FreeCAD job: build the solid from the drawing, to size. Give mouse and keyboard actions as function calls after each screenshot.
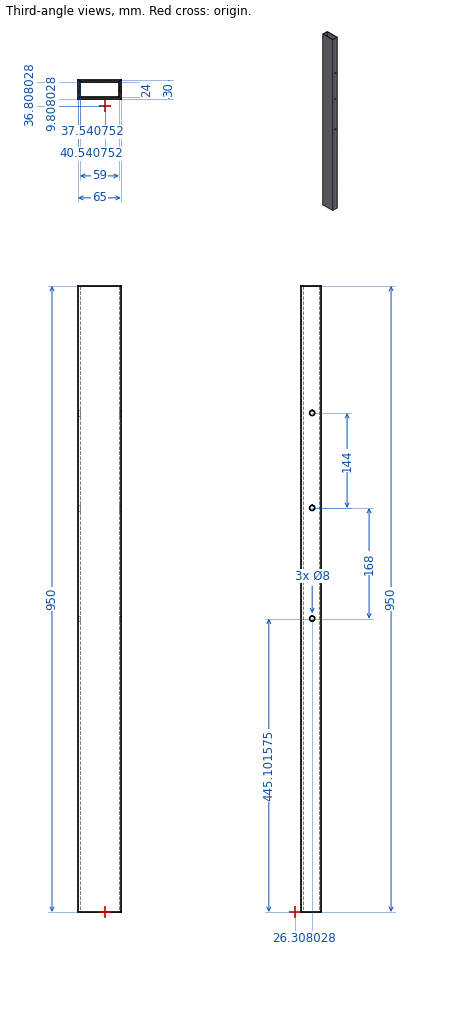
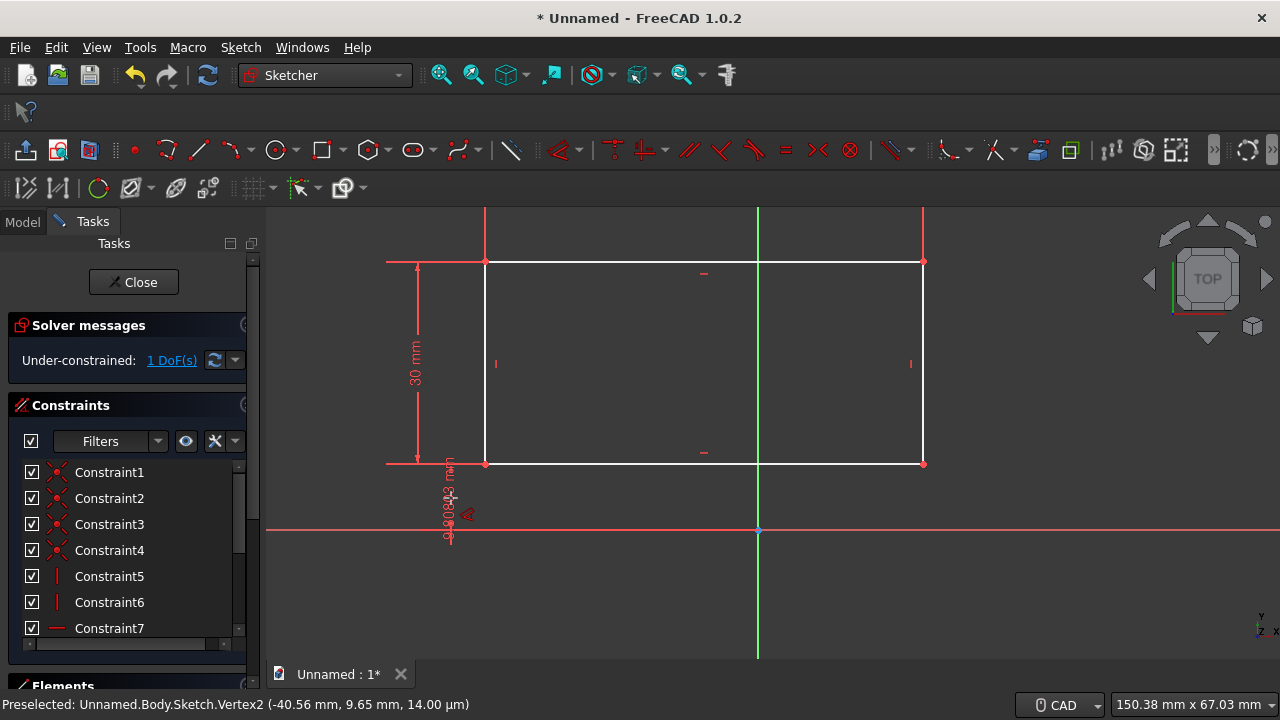
click(485, 262)
click(622, 564)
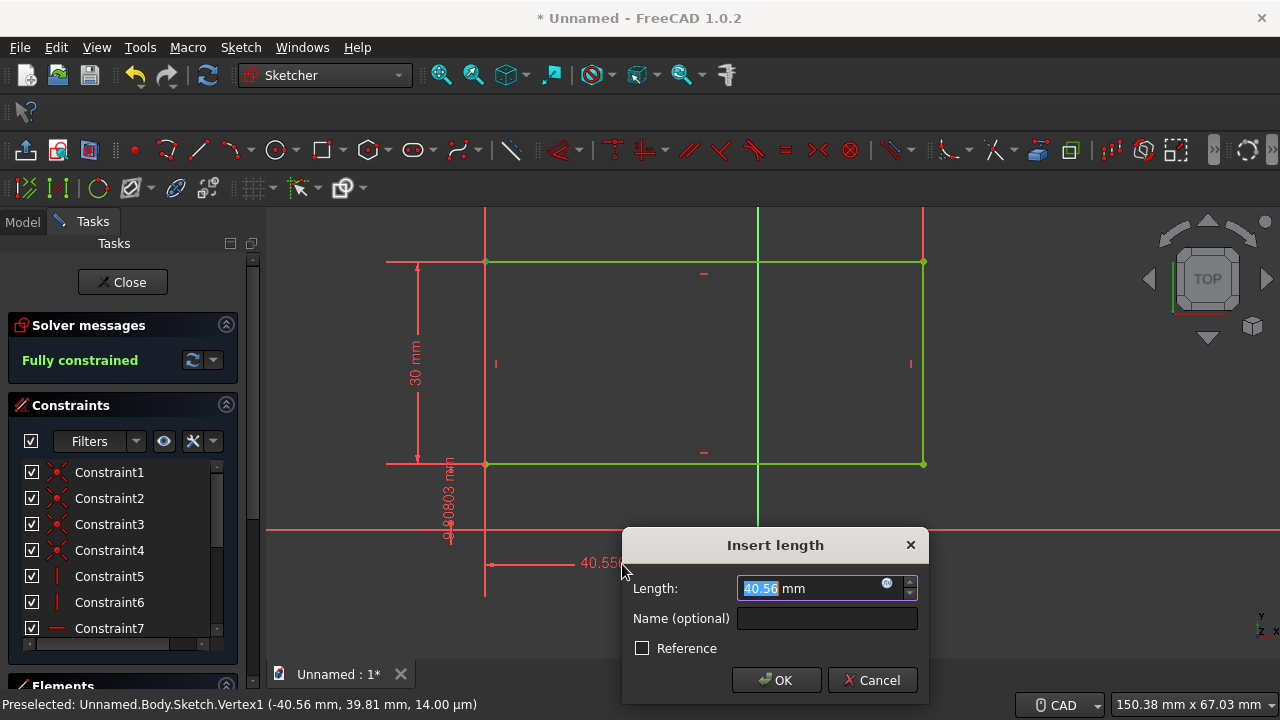
text(40.540752)
key(Return)
key(Escape)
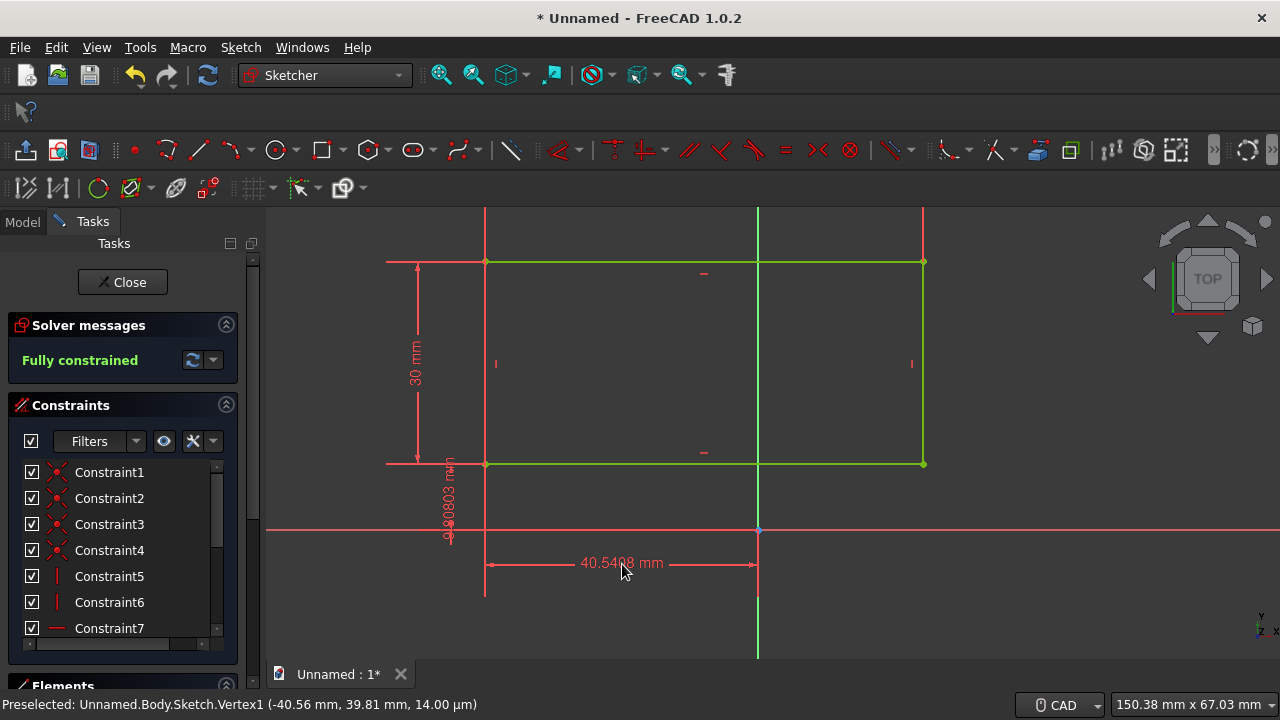
click(123, 282)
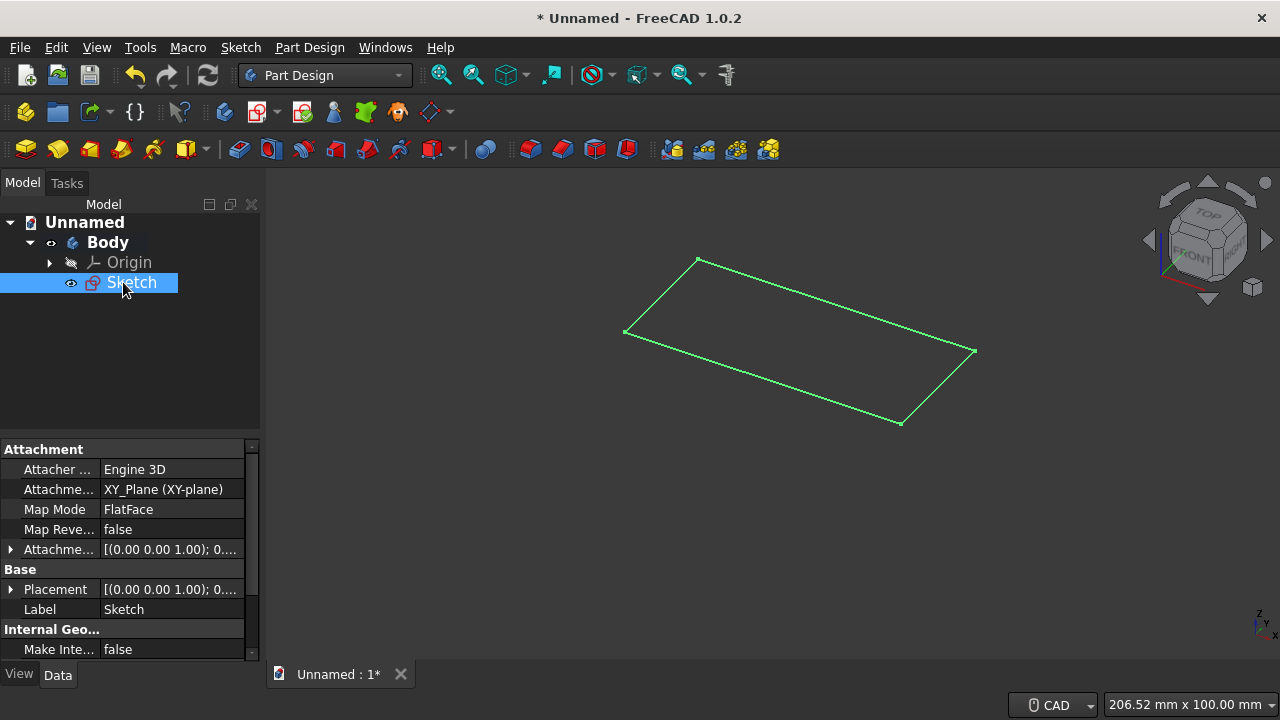
click(26, 150)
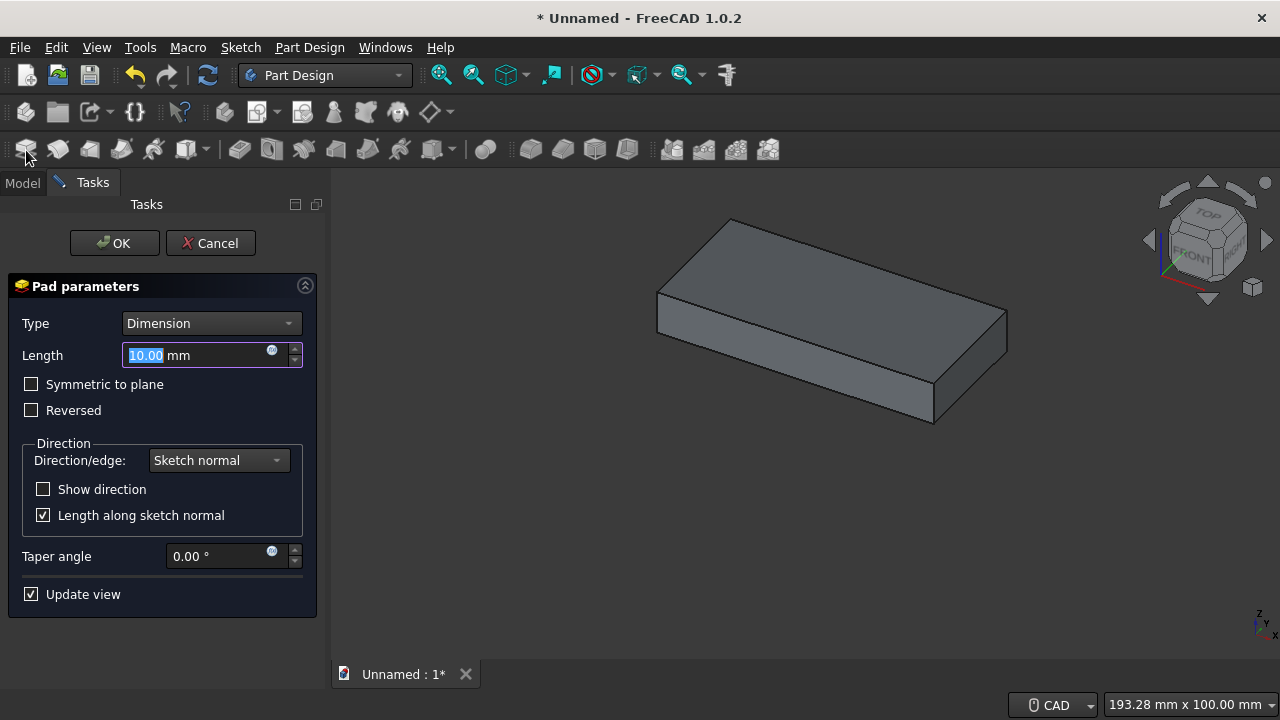
text(950)
key(Tab)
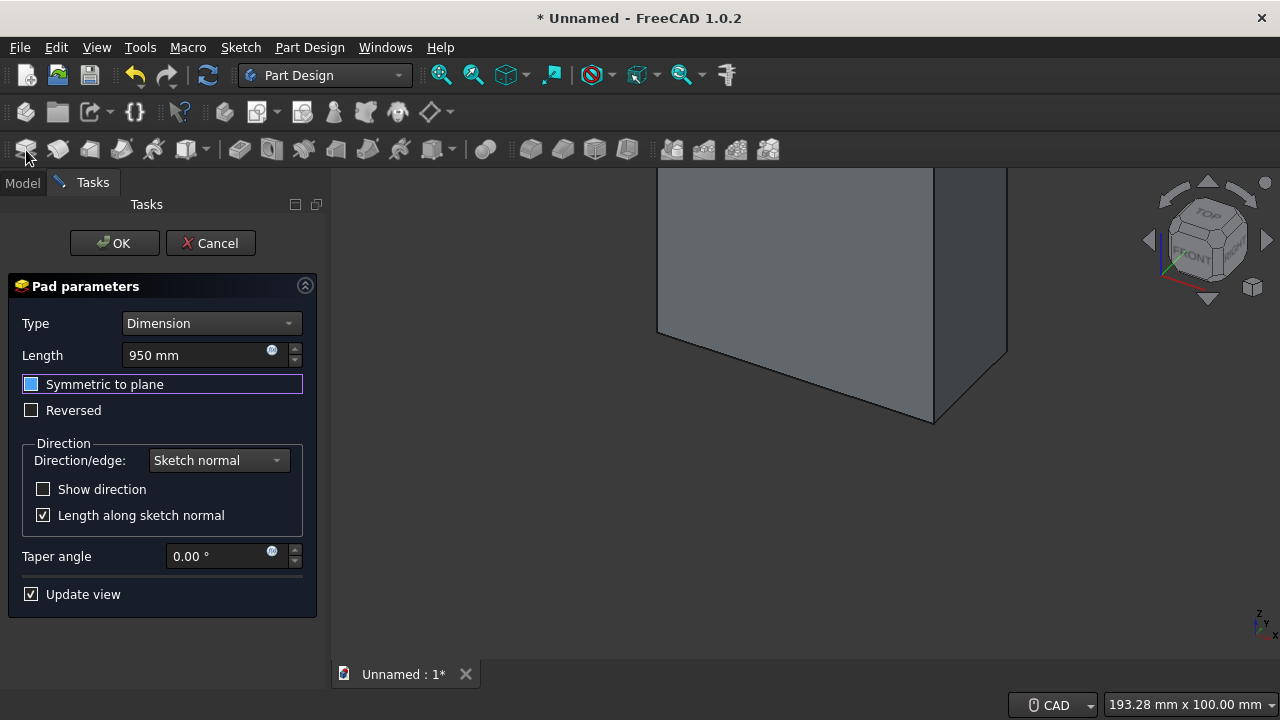
click(115, 243)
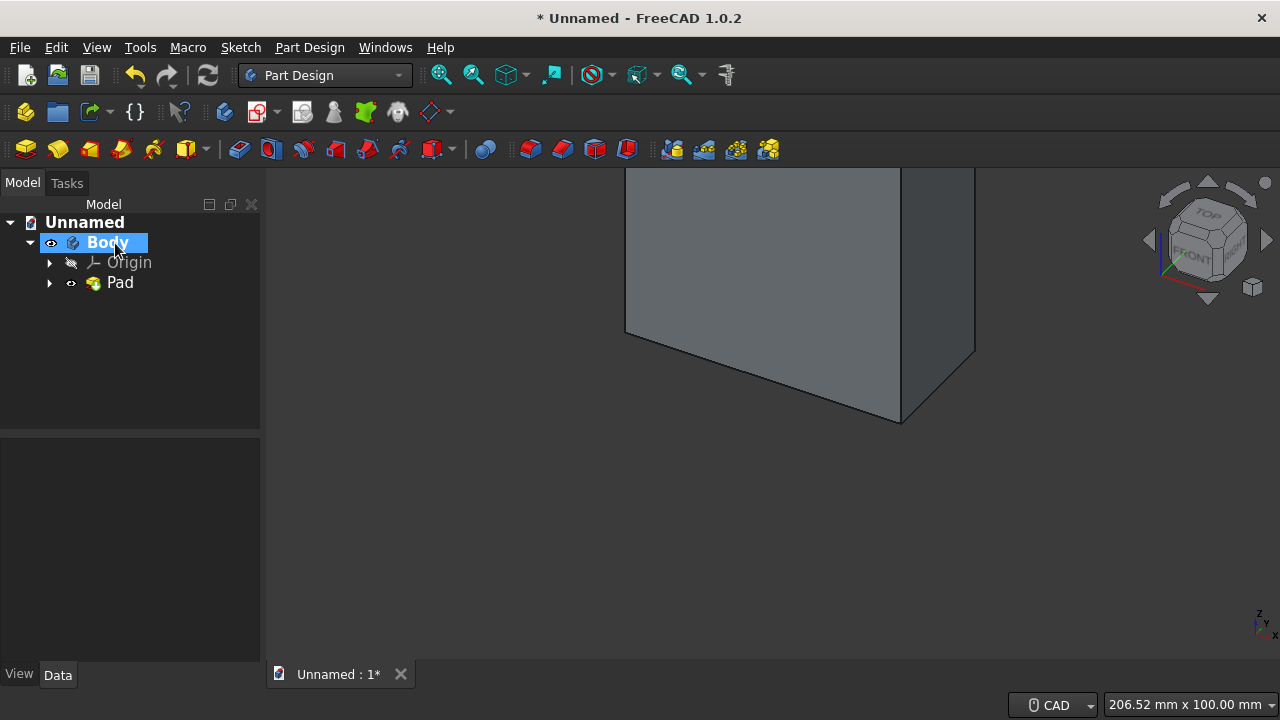
click(442, 76)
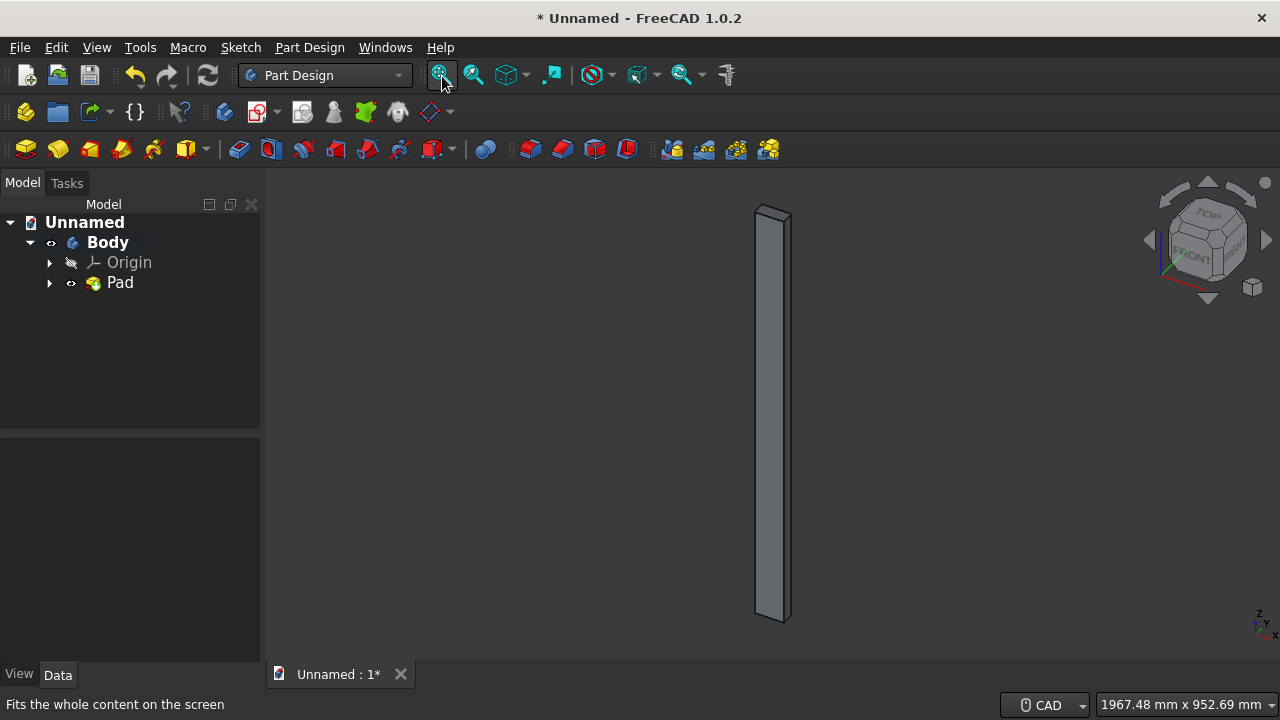
key(0)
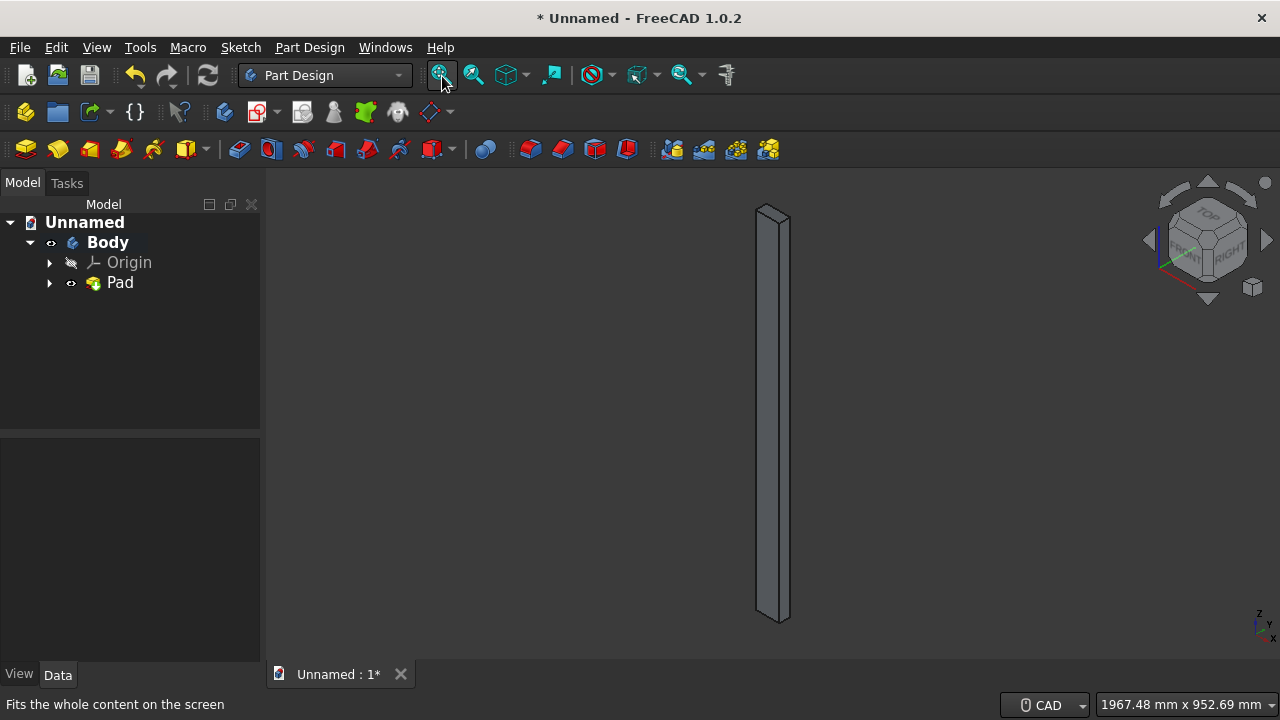
key(2)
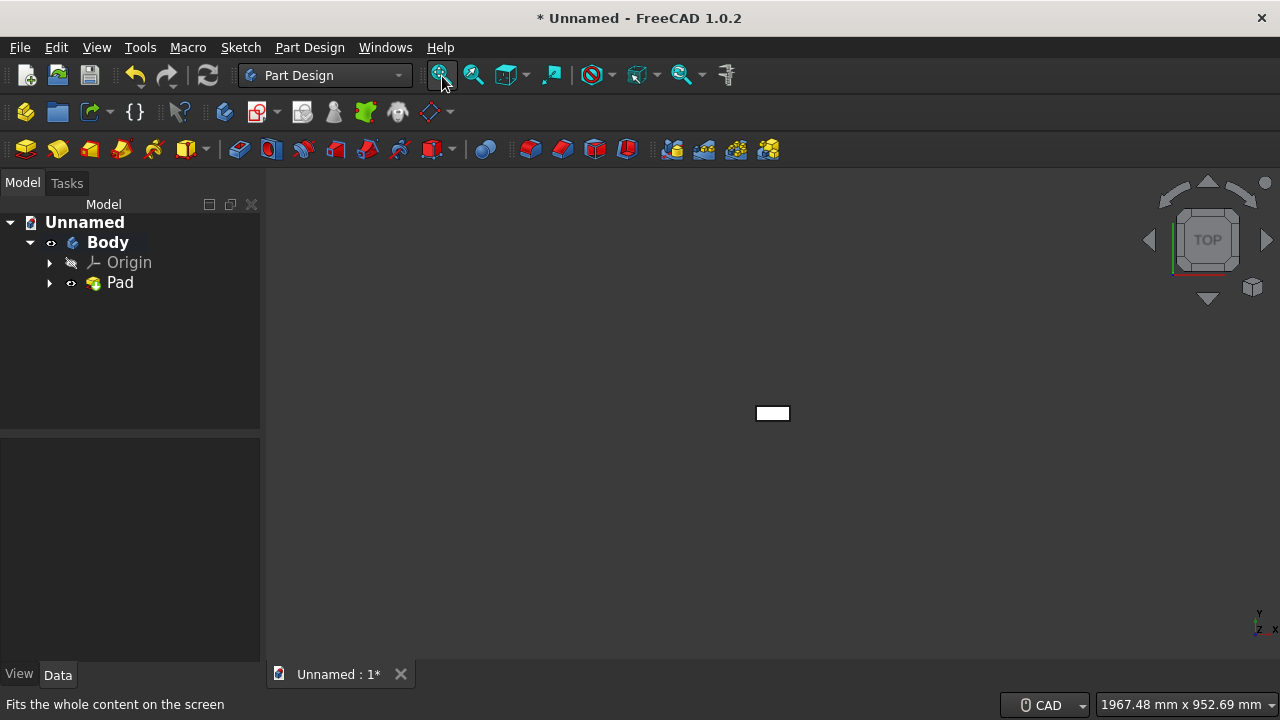
click(442, 76)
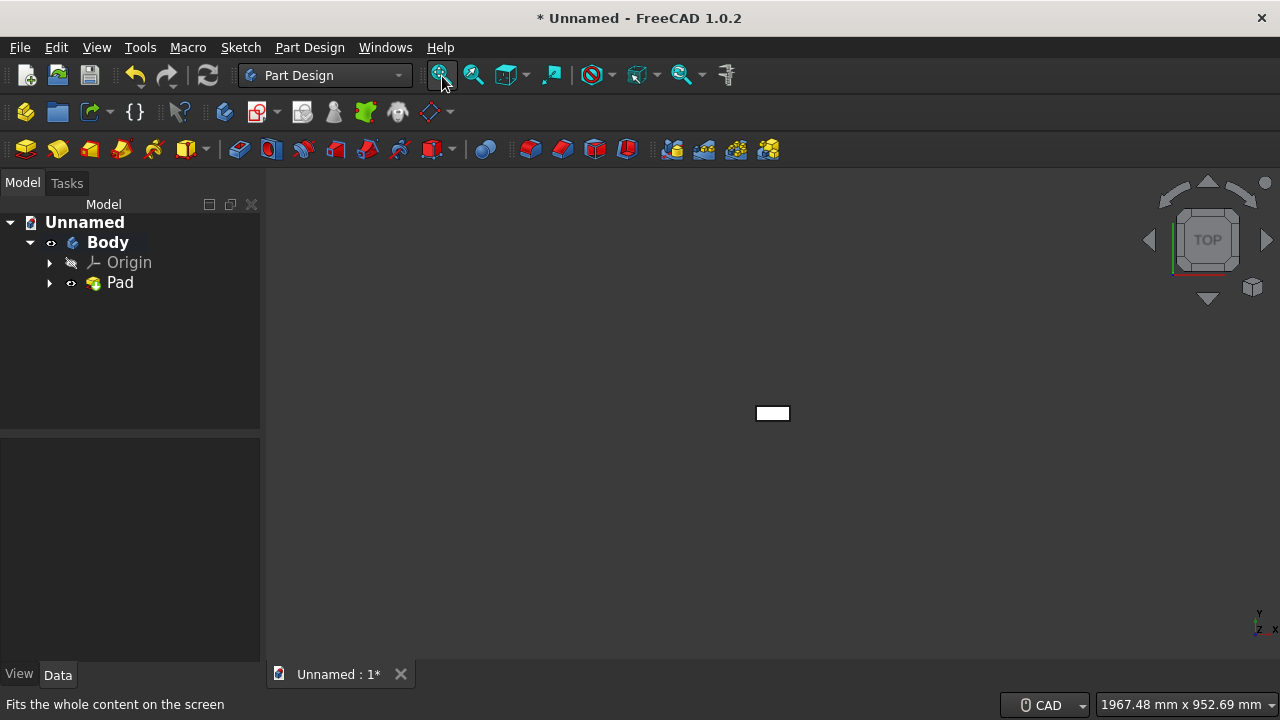
key(1)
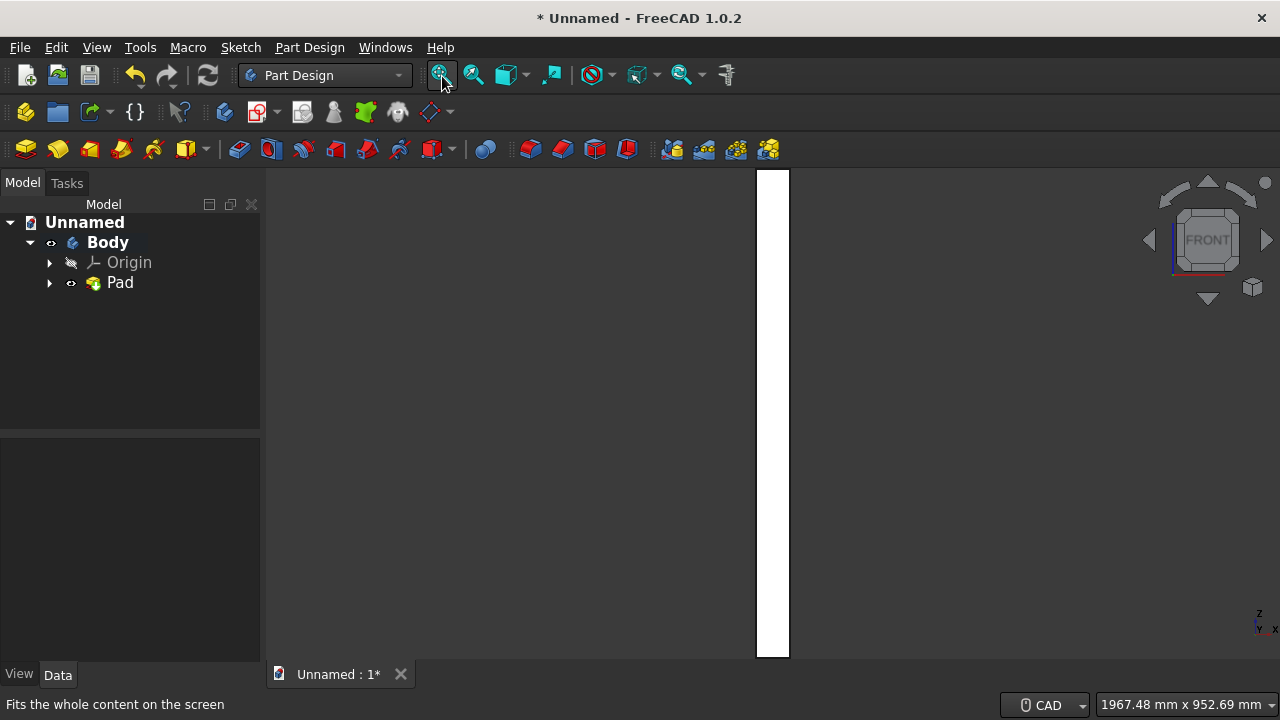
click(50, 263)